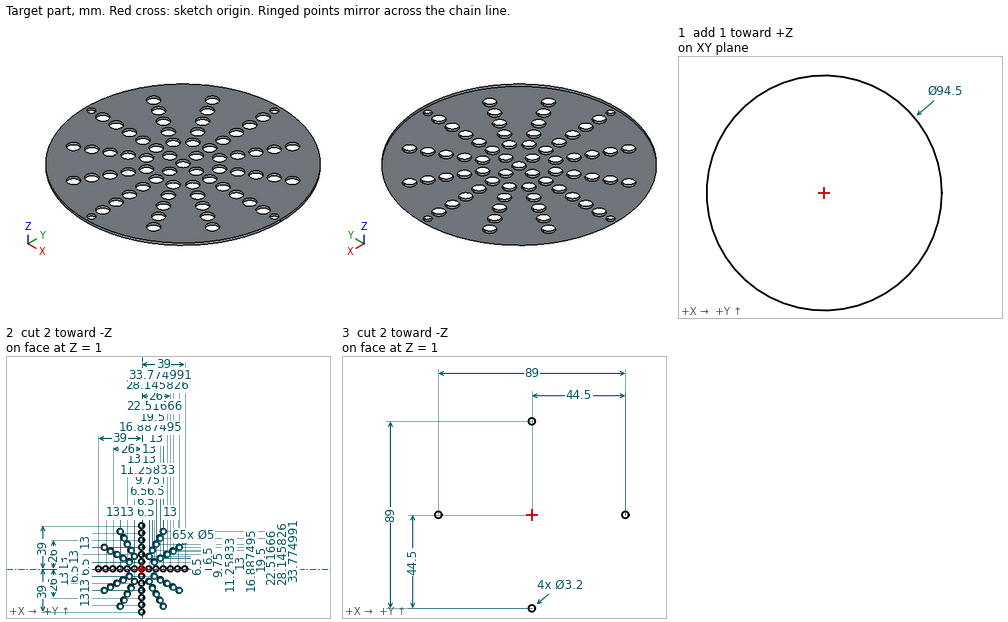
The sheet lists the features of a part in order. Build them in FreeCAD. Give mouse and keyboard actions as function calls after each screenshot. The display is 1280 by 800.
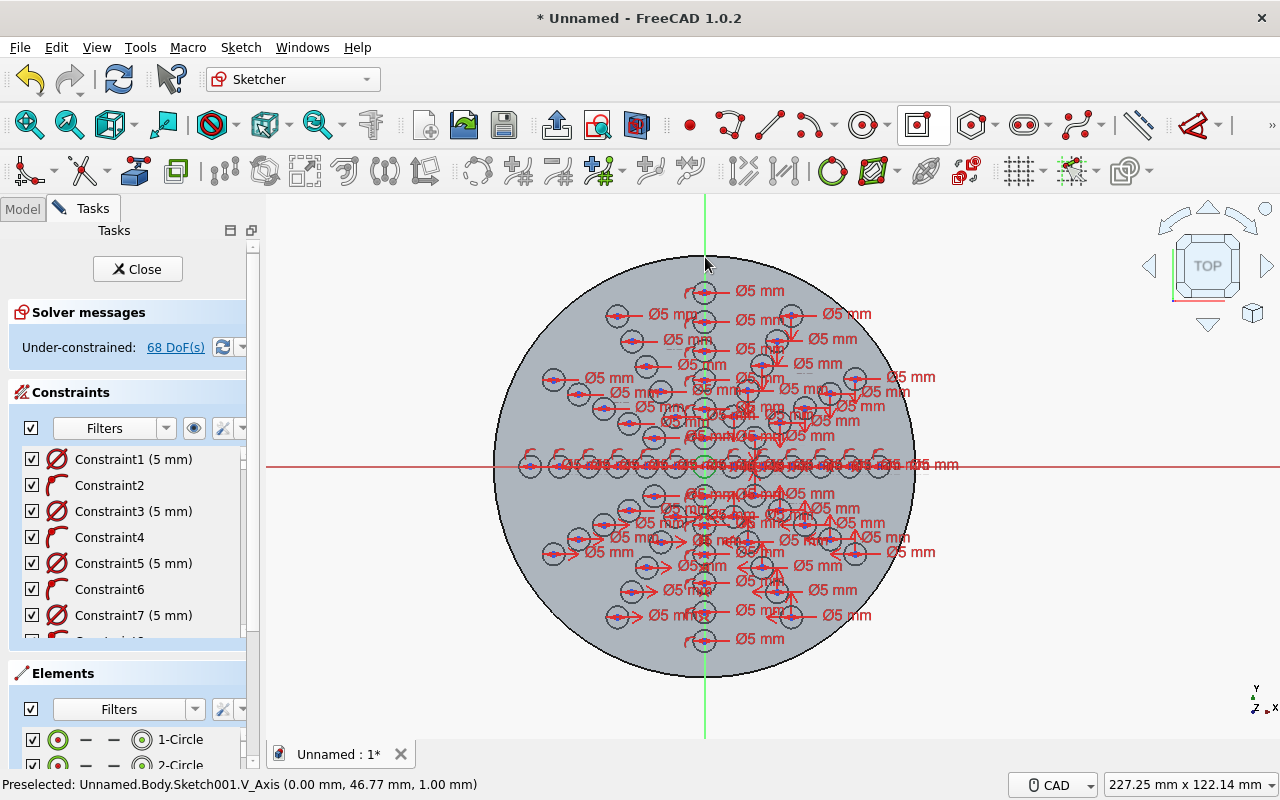
click(780, 510)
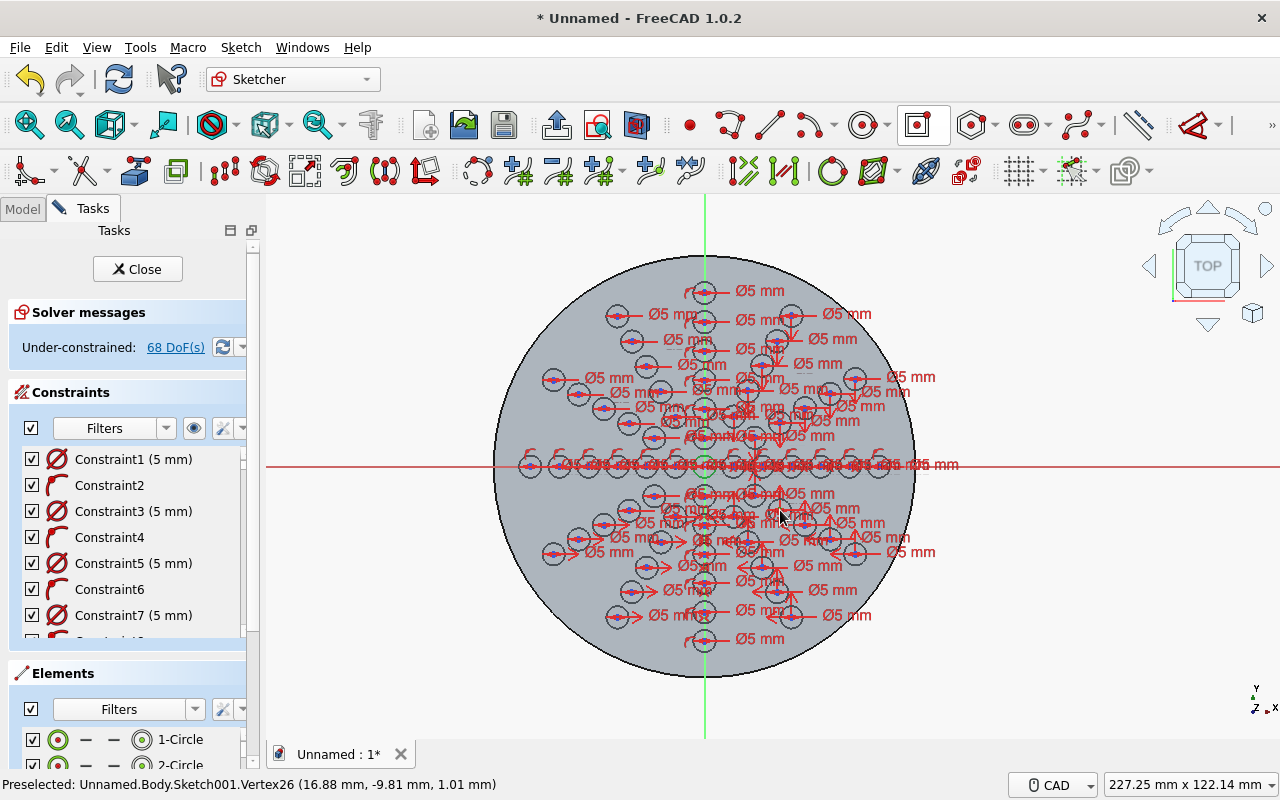
click(629, 511)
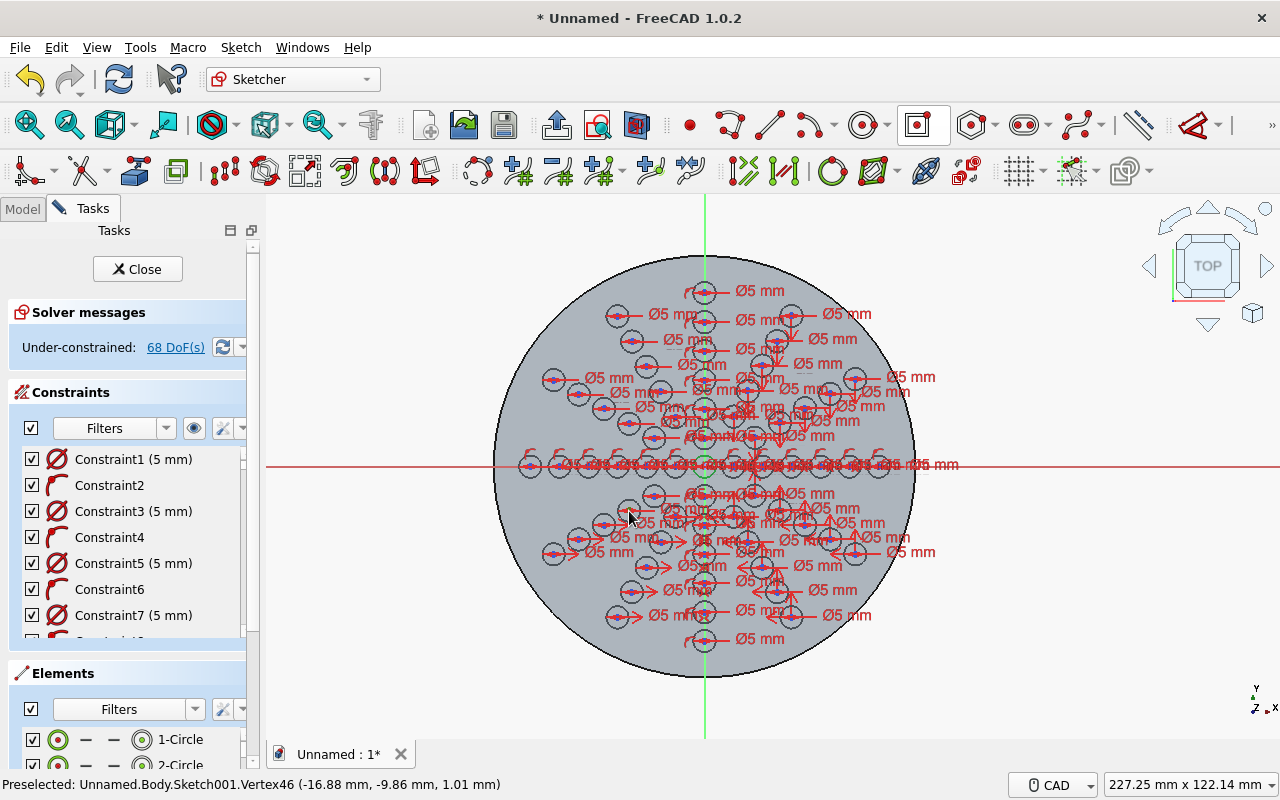
click(705, 257)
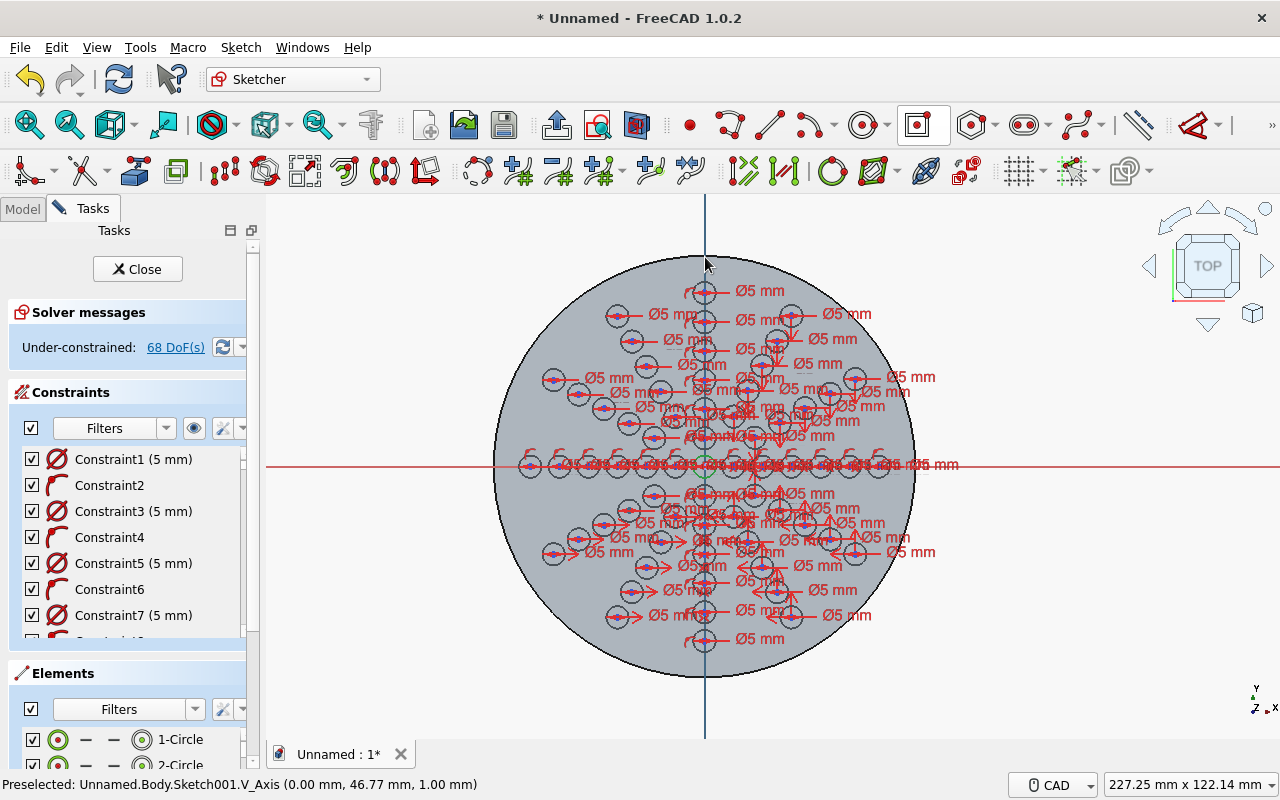
key(s)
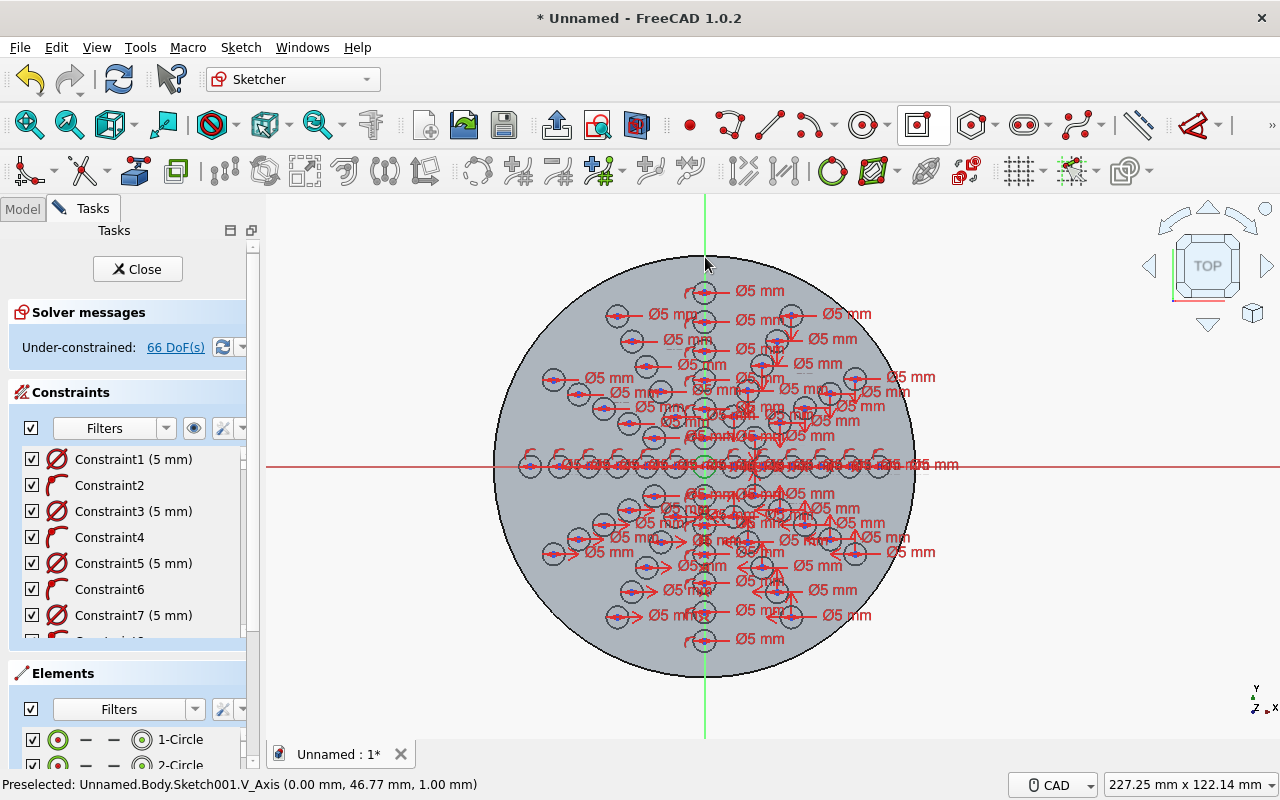
click(755, 496)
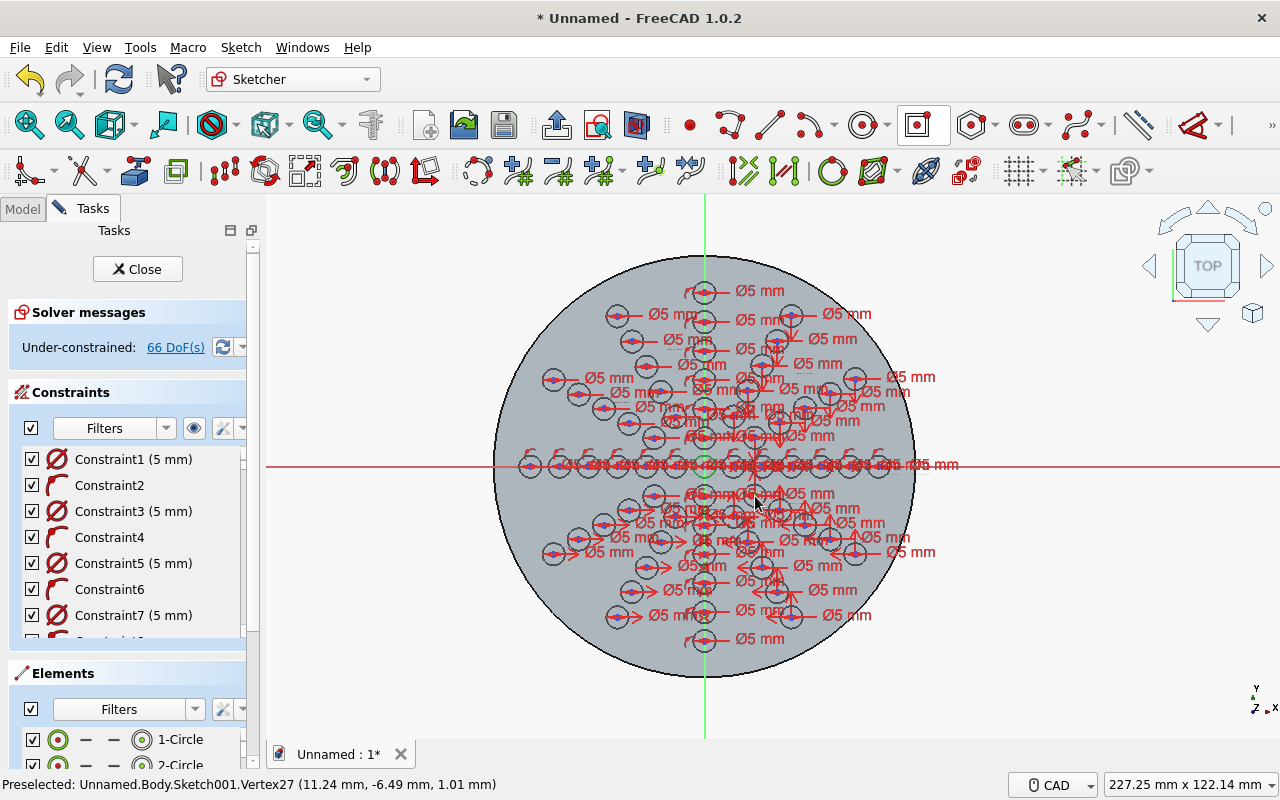
click(654, 496)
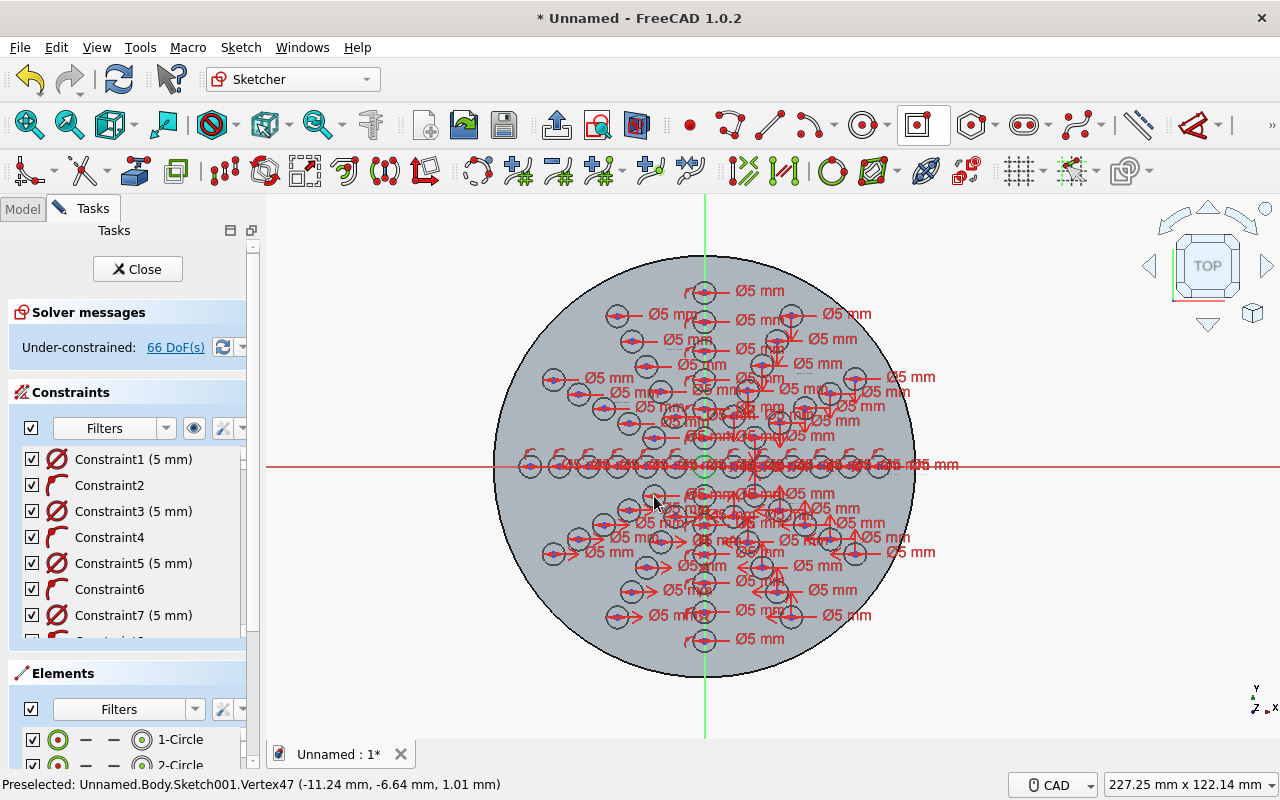
click(705, 257)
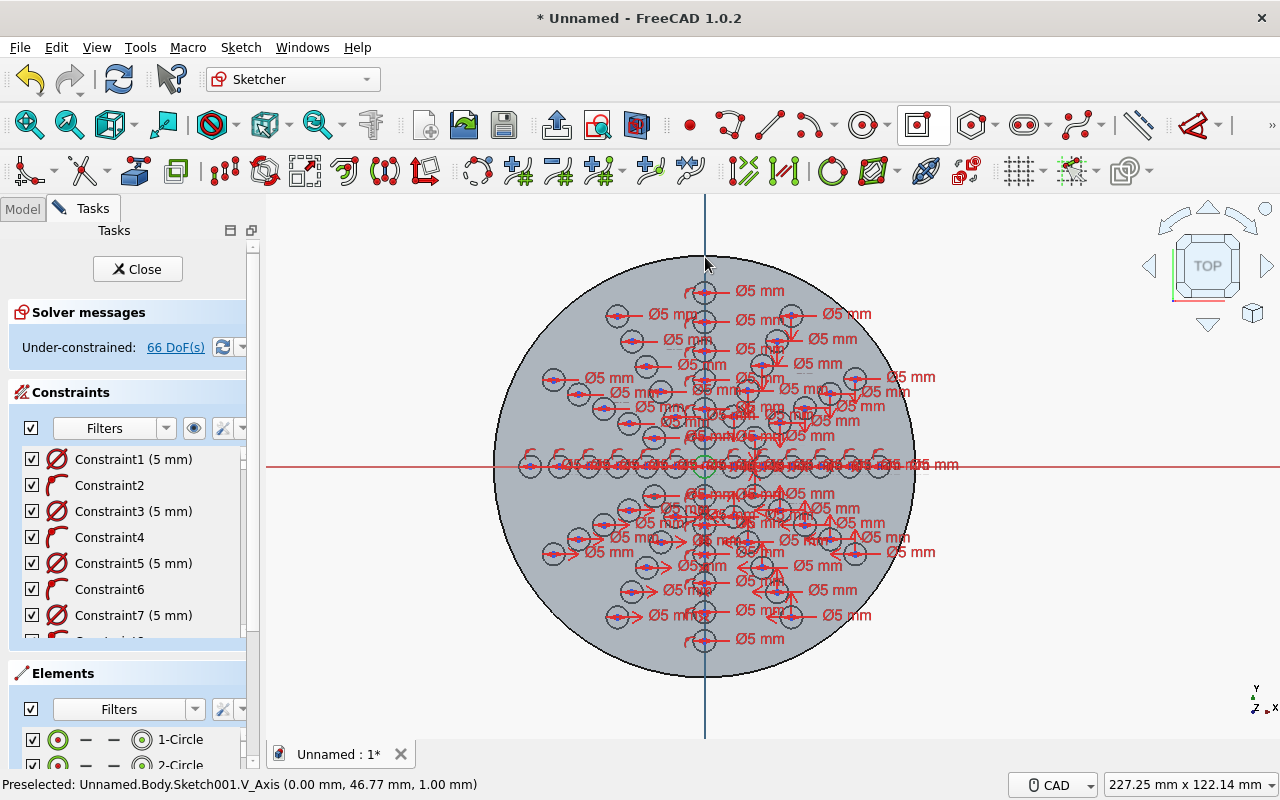
key(s)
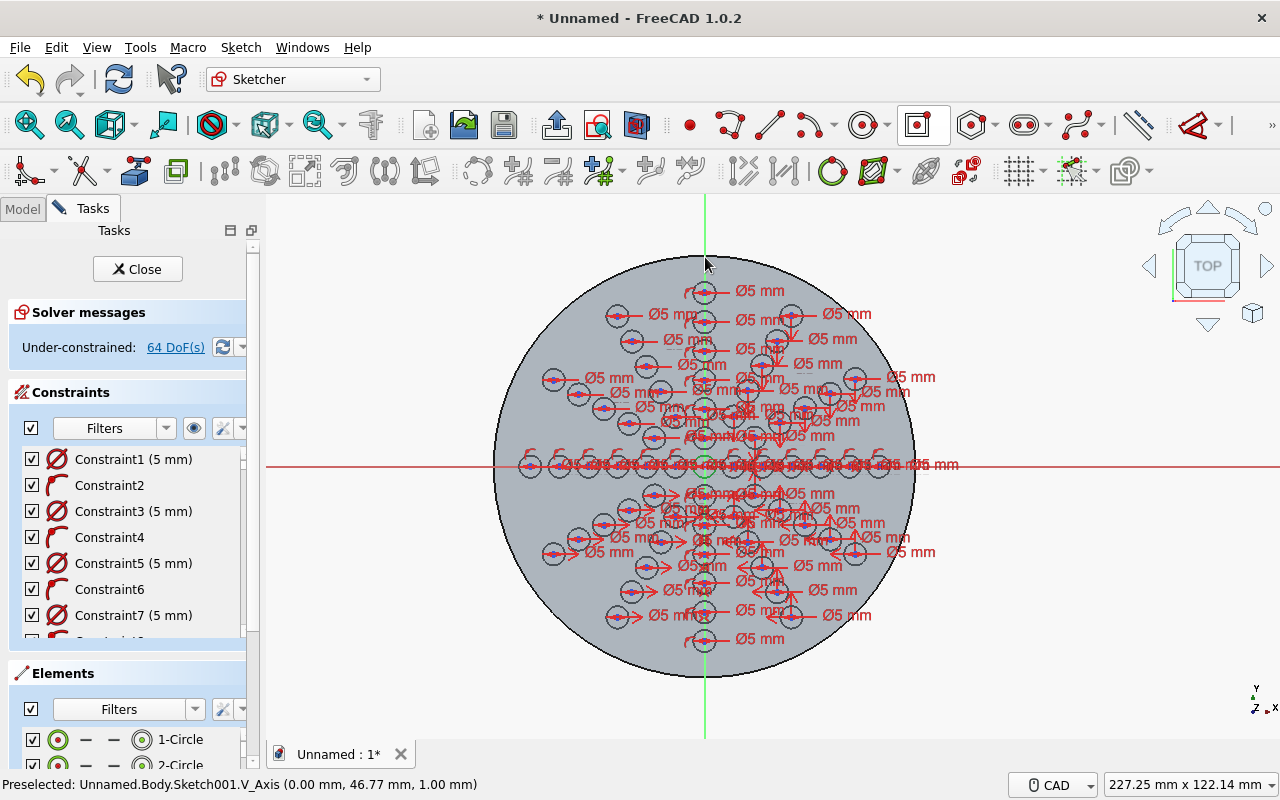
click(855, 379)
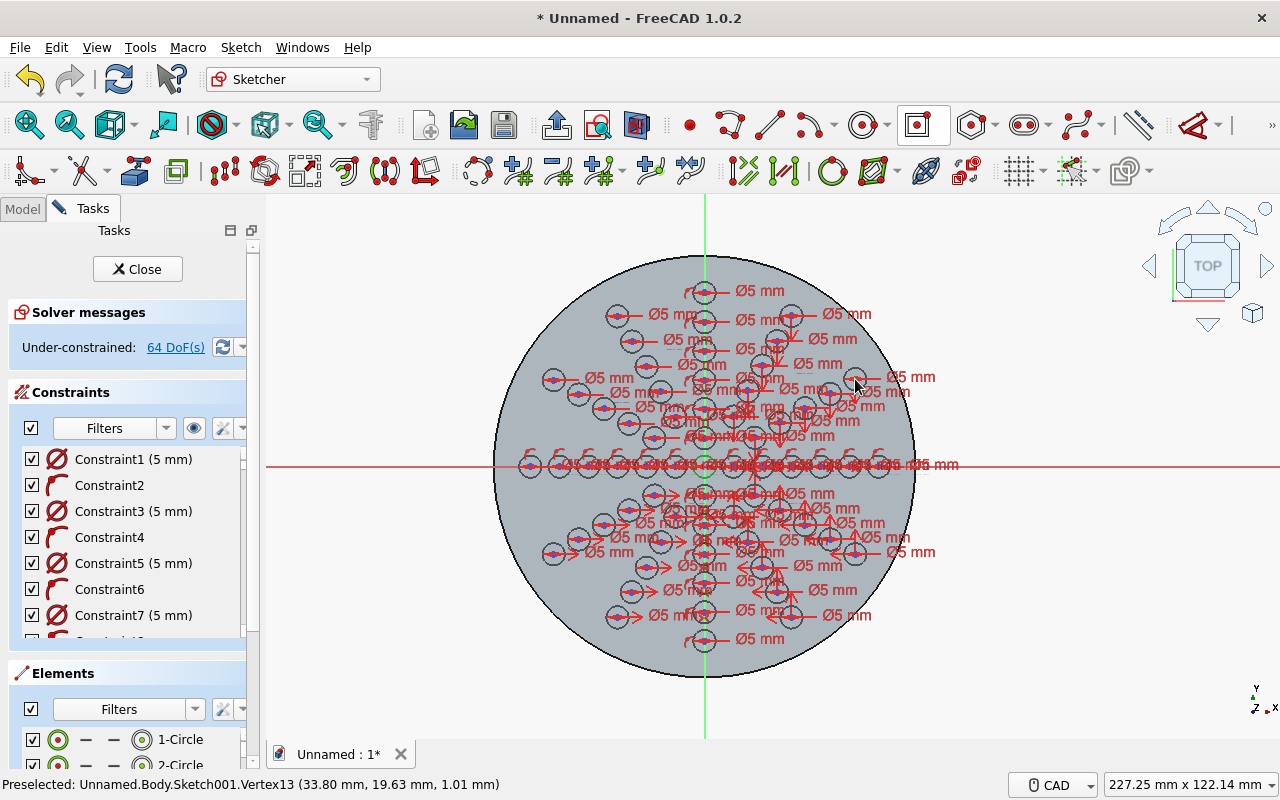
click(554, 380)